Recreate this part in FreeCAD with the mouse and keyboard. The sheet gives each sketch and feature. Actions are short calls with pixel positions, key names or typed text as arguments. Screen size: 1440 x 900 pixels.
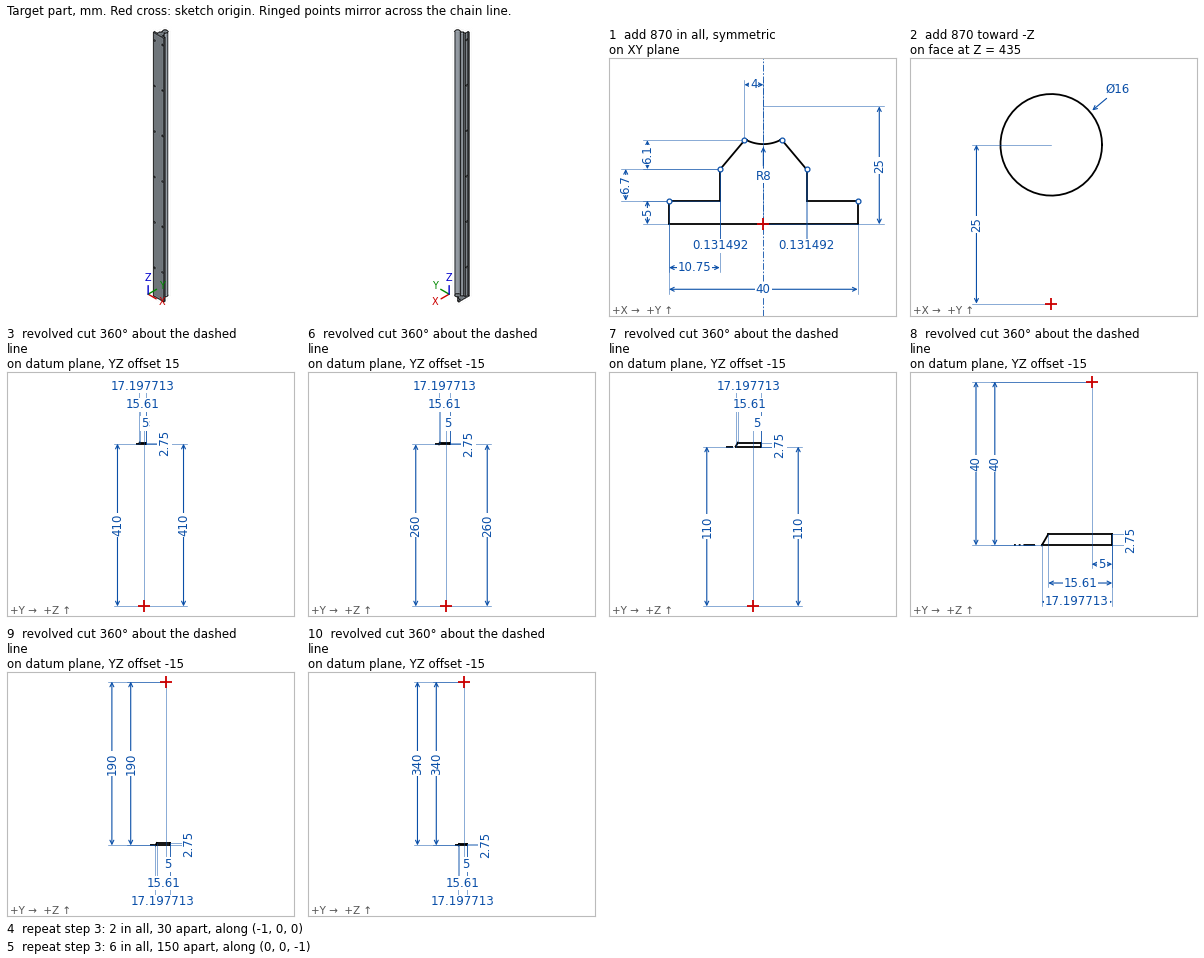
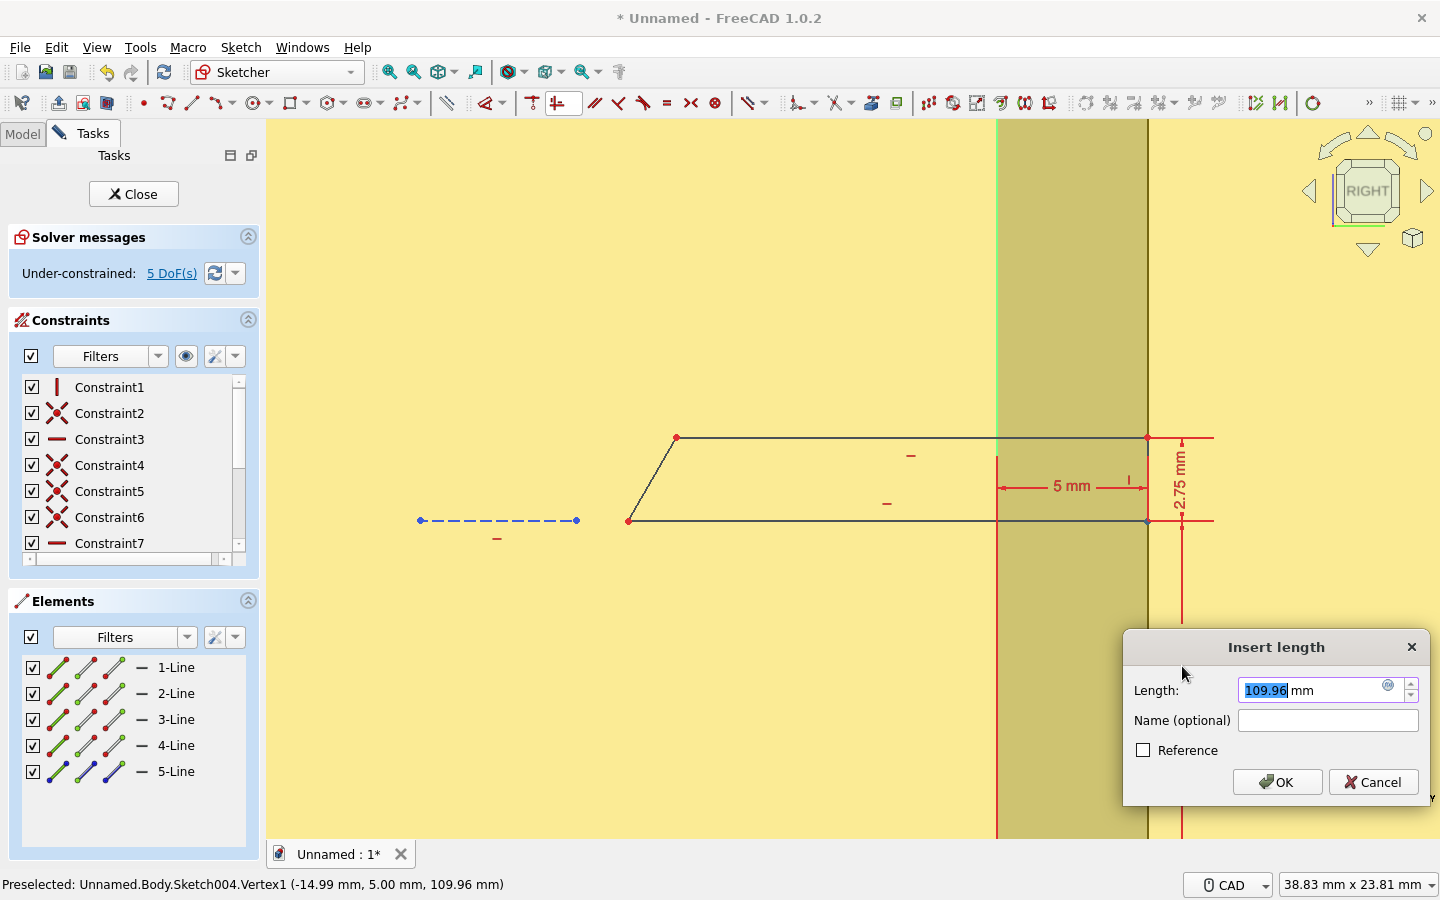
text(110)
key(Return)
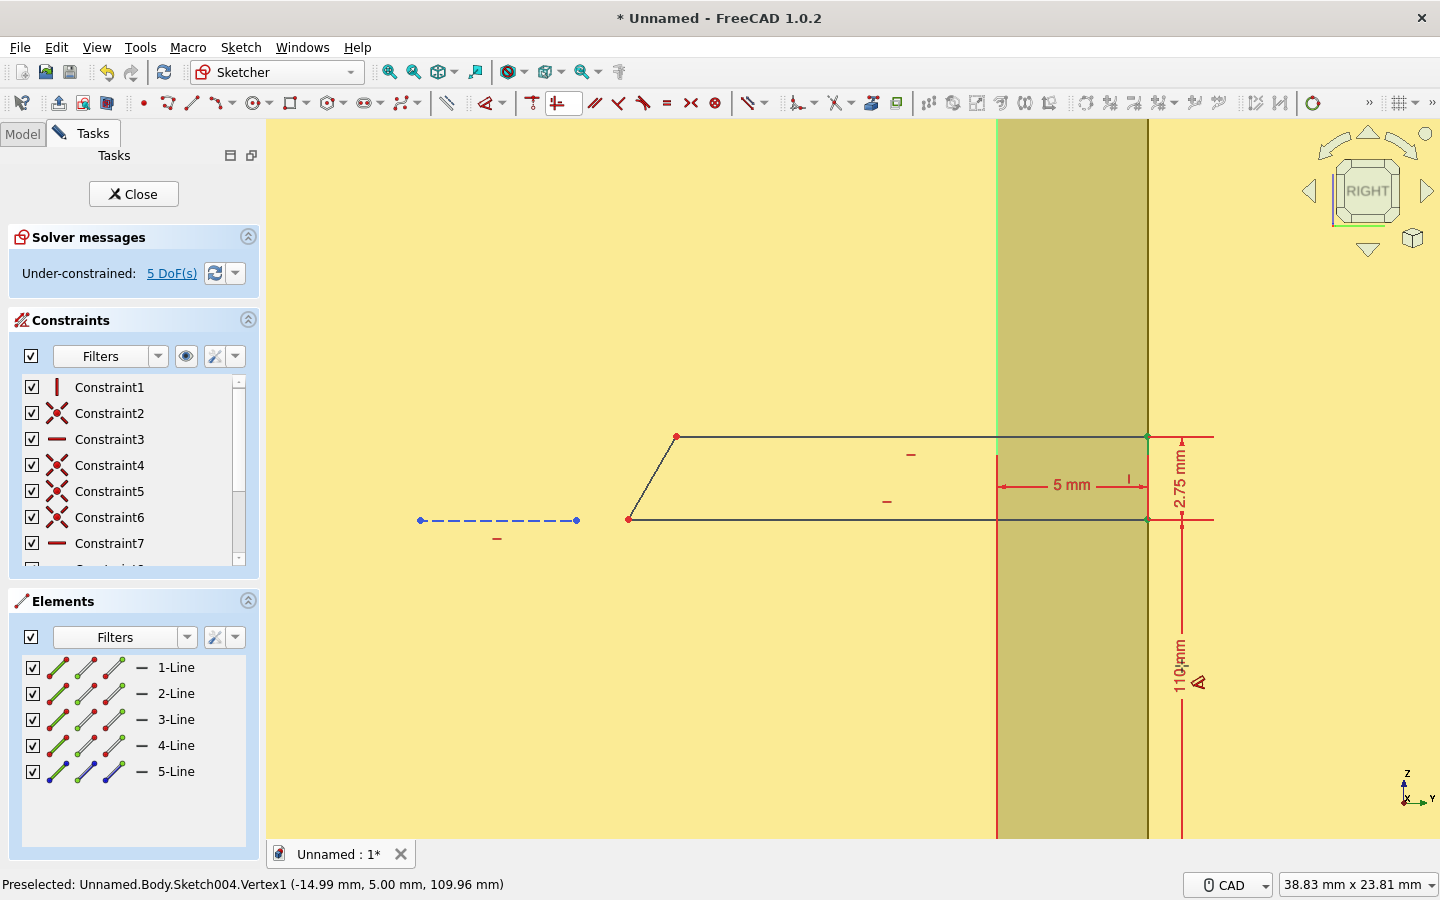
click(576, 521)
click(1031, 666)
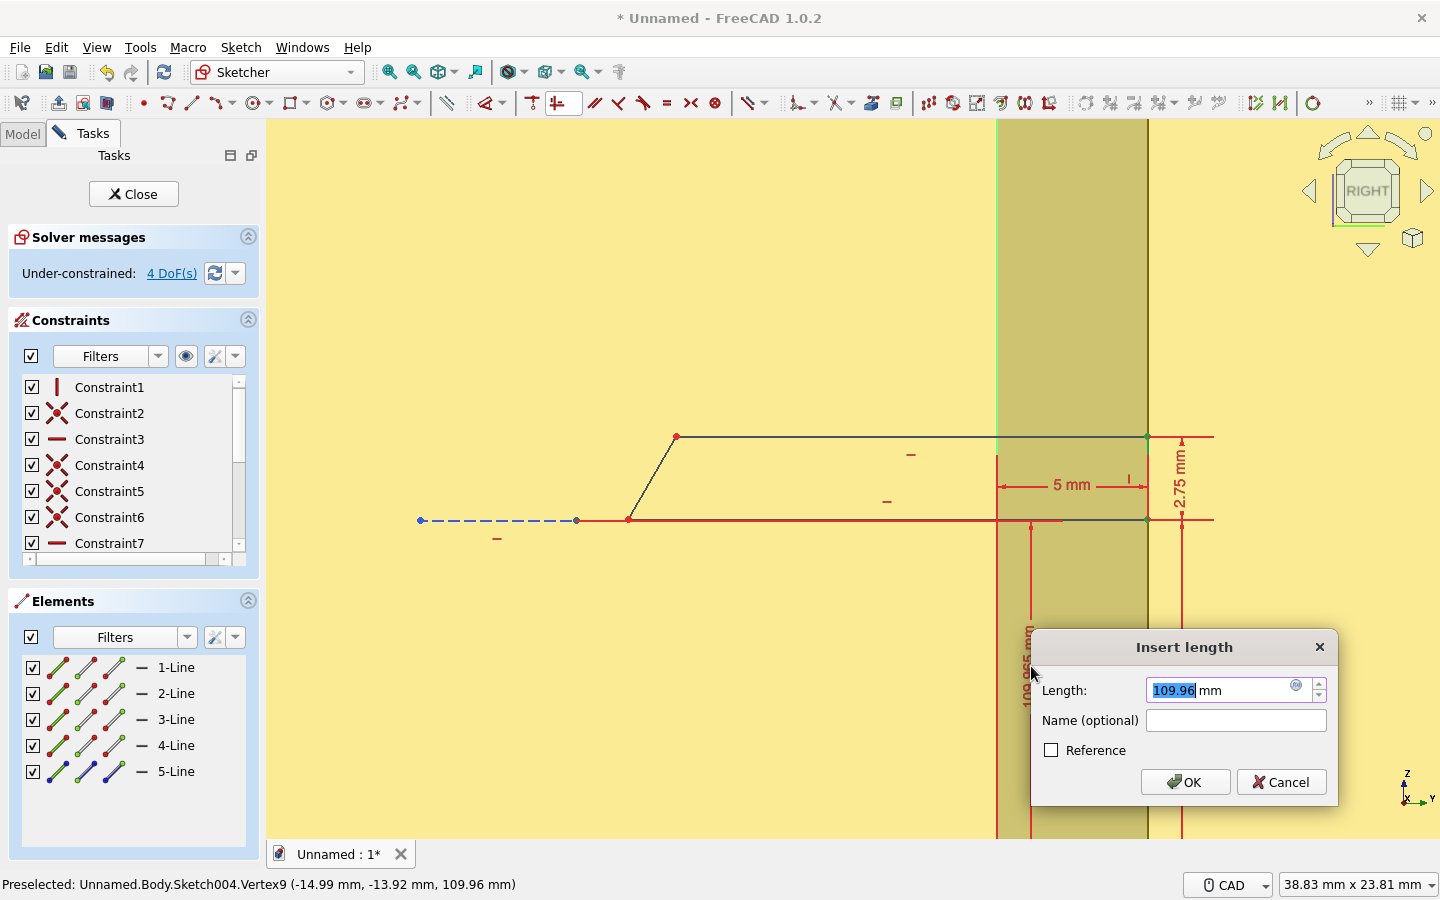
text(110)
key(Return)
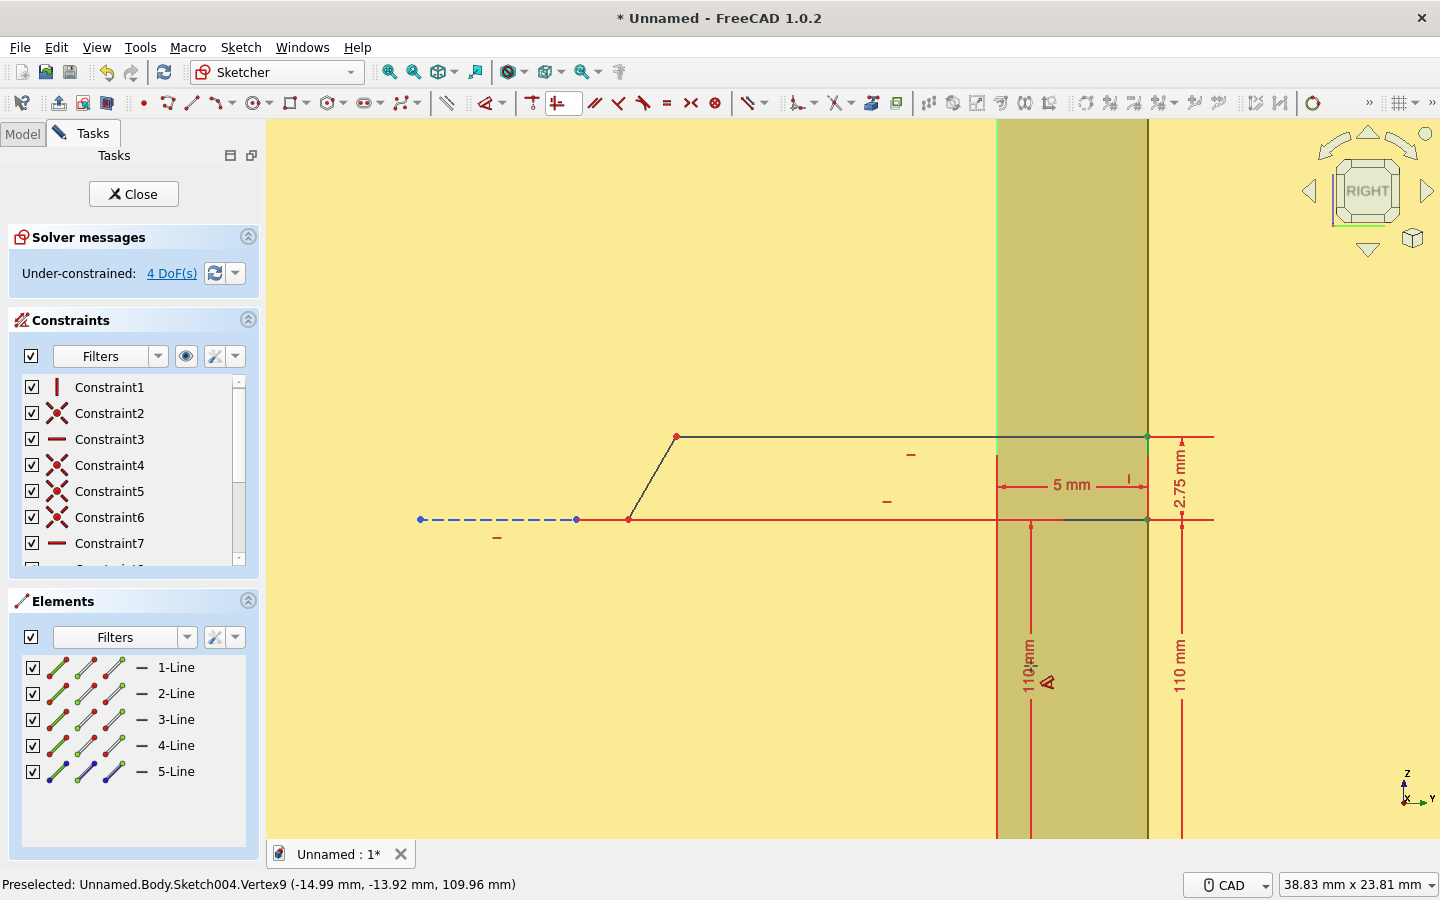
scroll(1006, 437, up, 2)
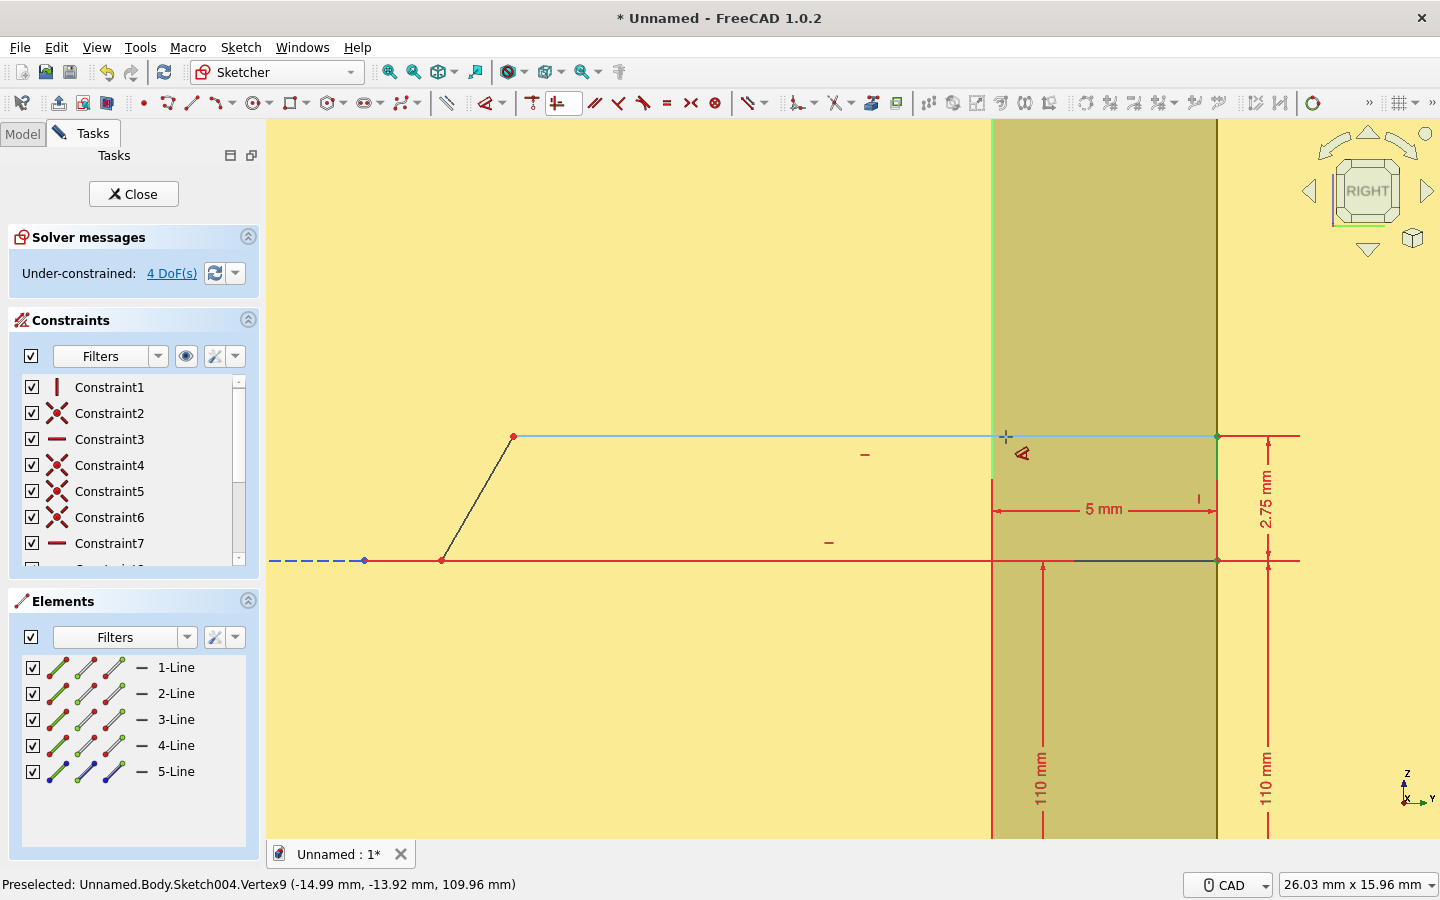
click(1006, 436)
click(865, 402)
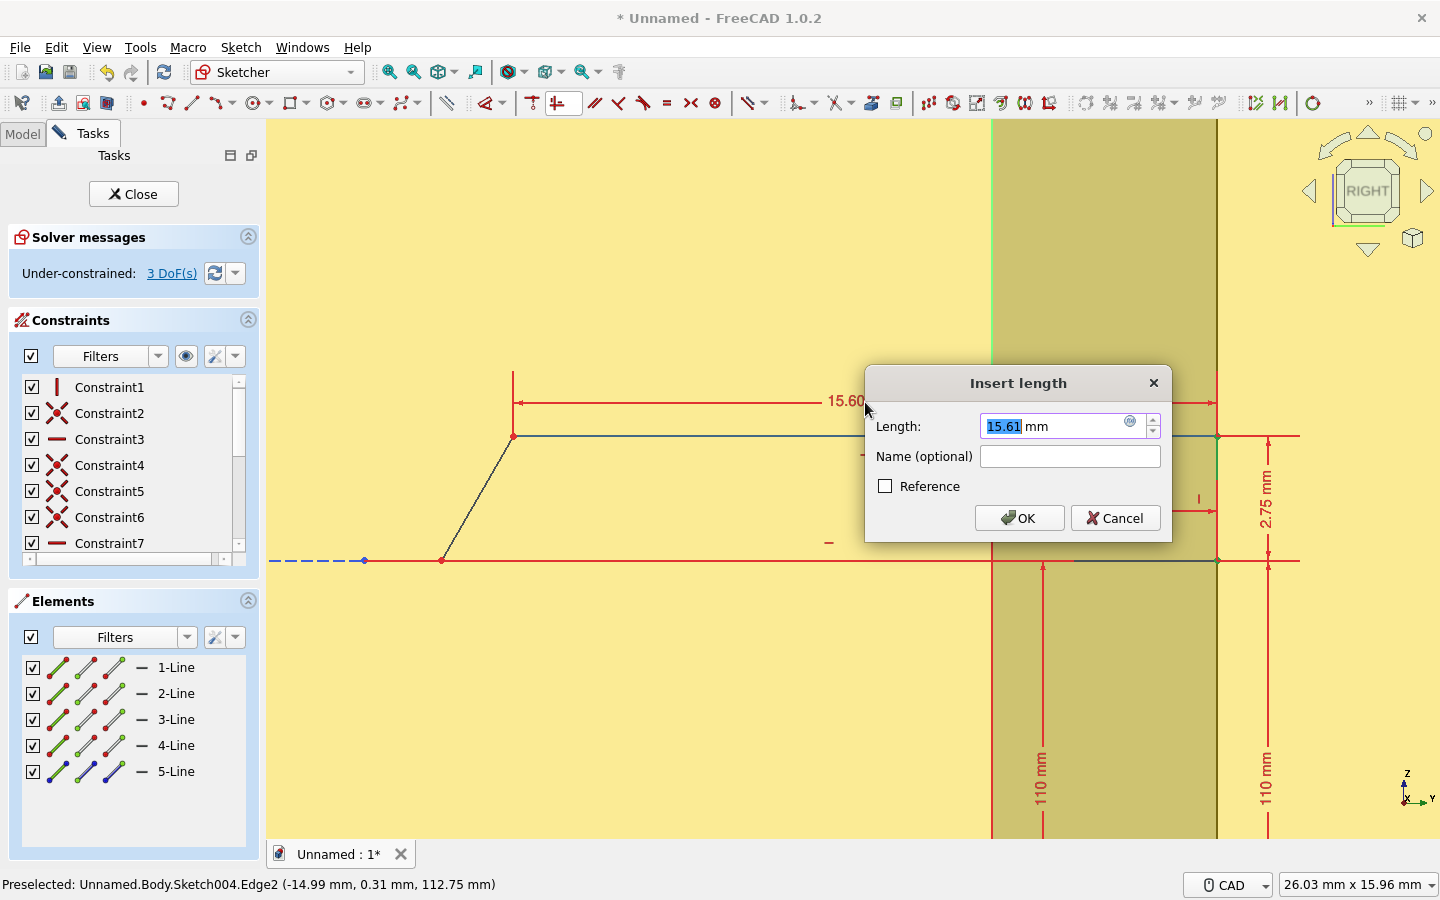
text(15.61)
key(Return)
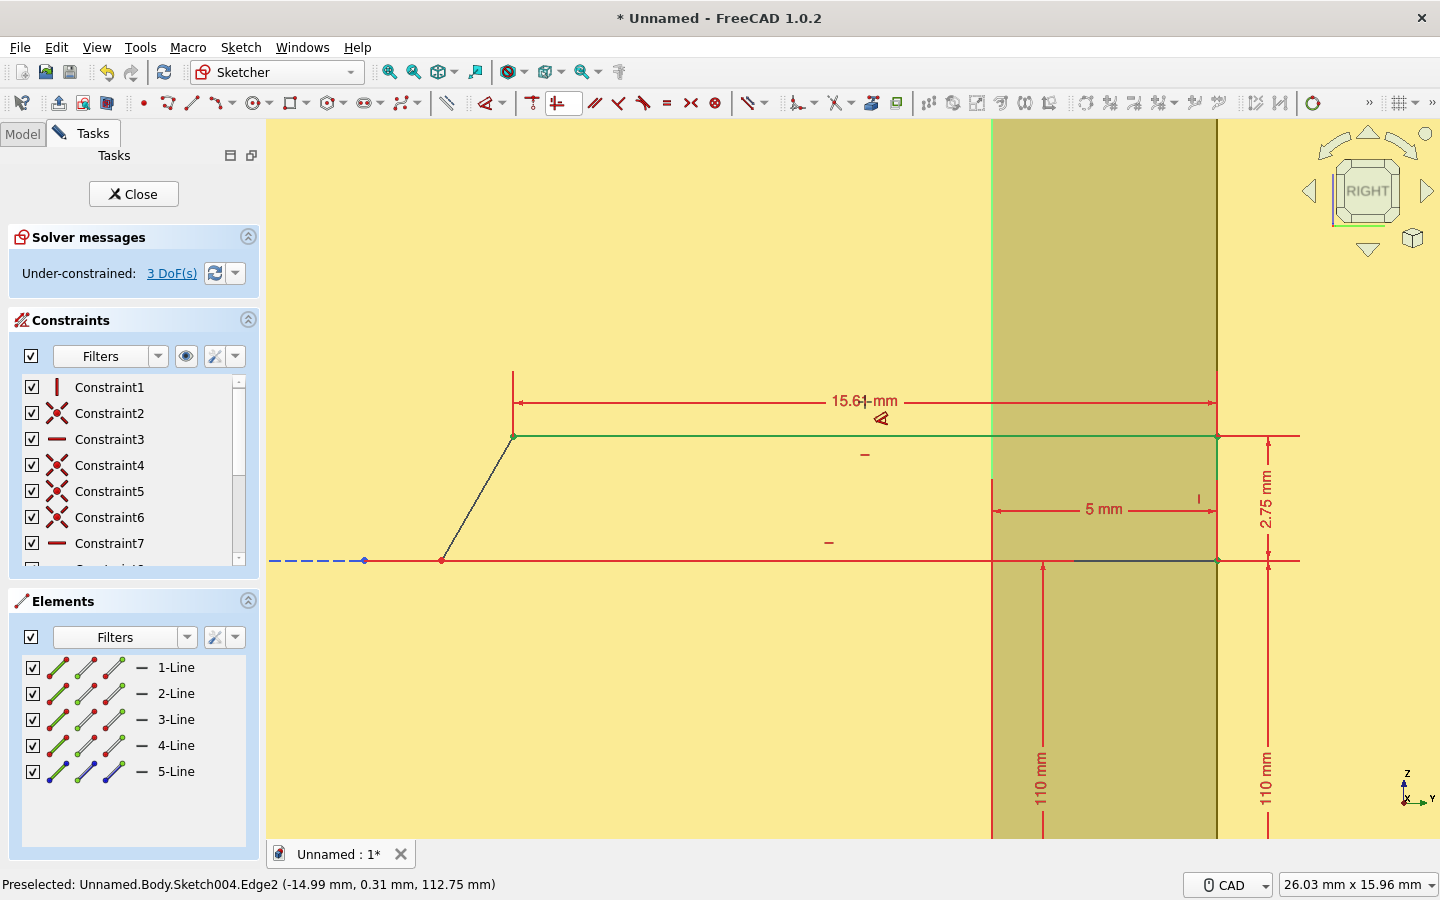
click(674, 561)
click(830, 595)